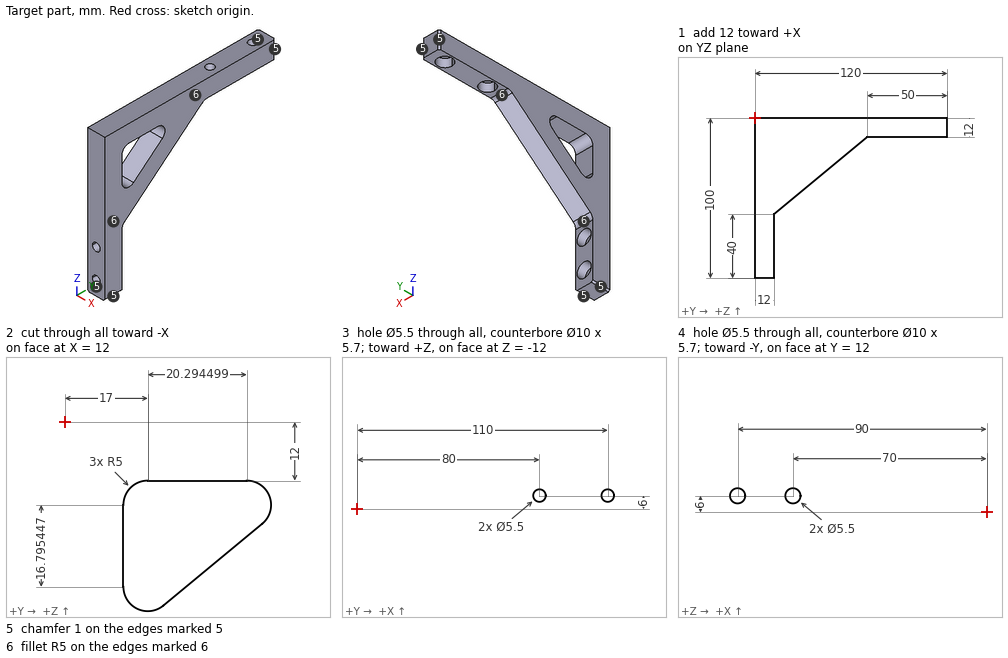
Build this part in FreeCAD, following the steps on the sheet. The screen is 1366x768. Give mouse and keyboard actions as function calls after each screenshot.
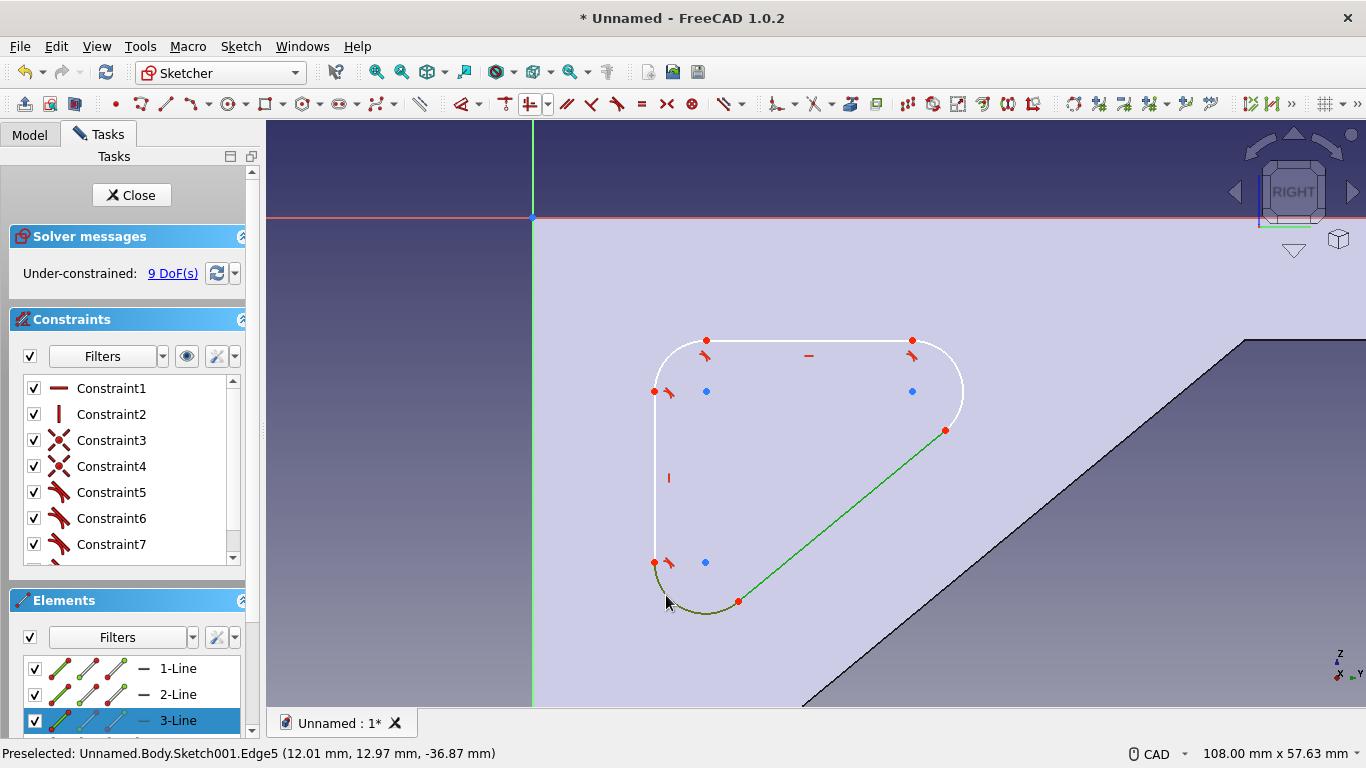
click(617, 104)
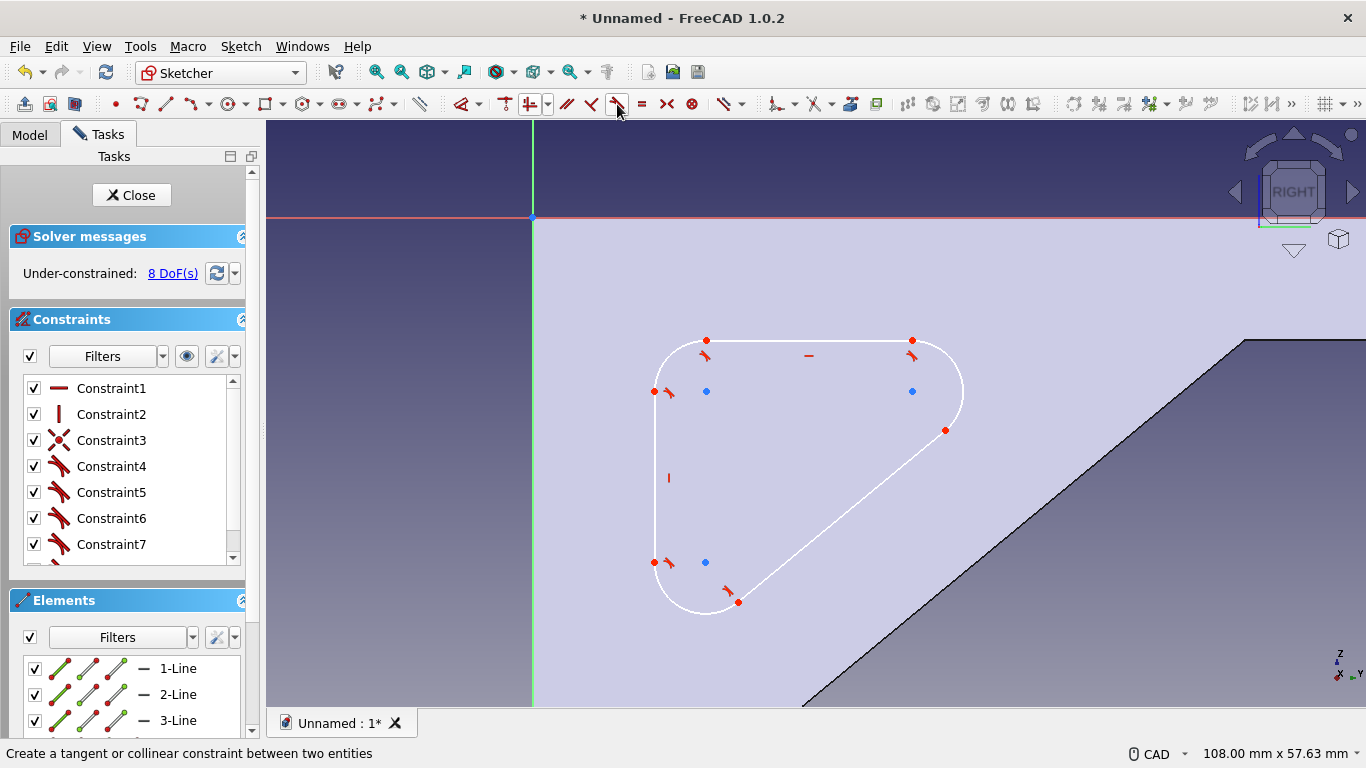
click(800, 551)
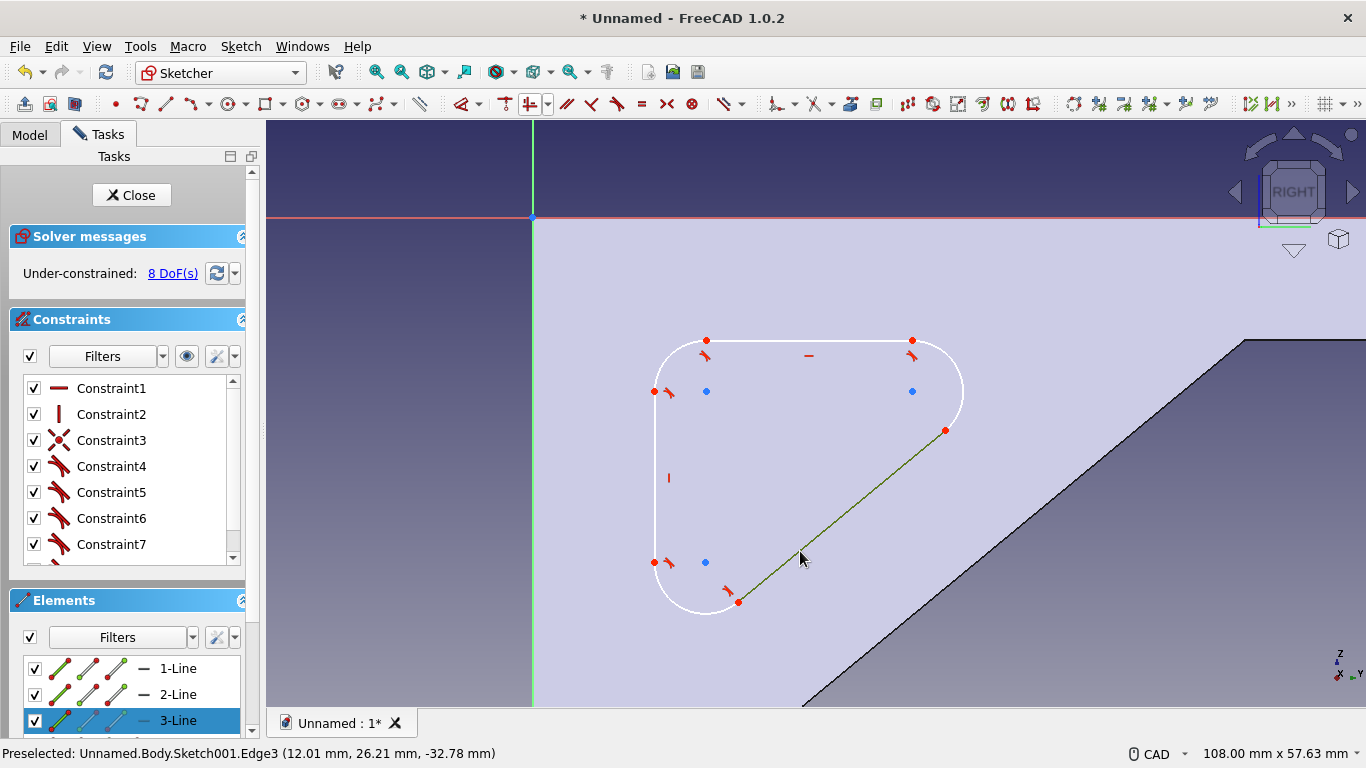
click(963, 399)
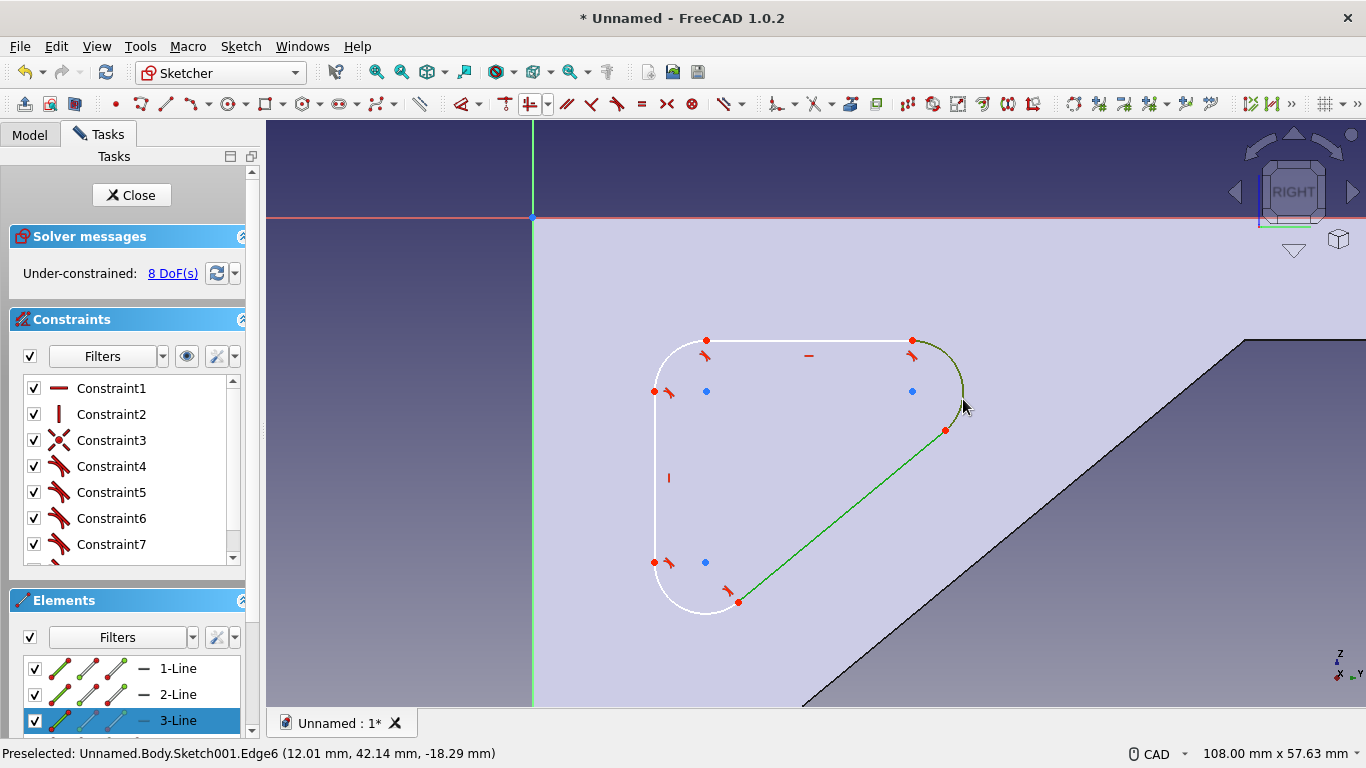
click(617, 104)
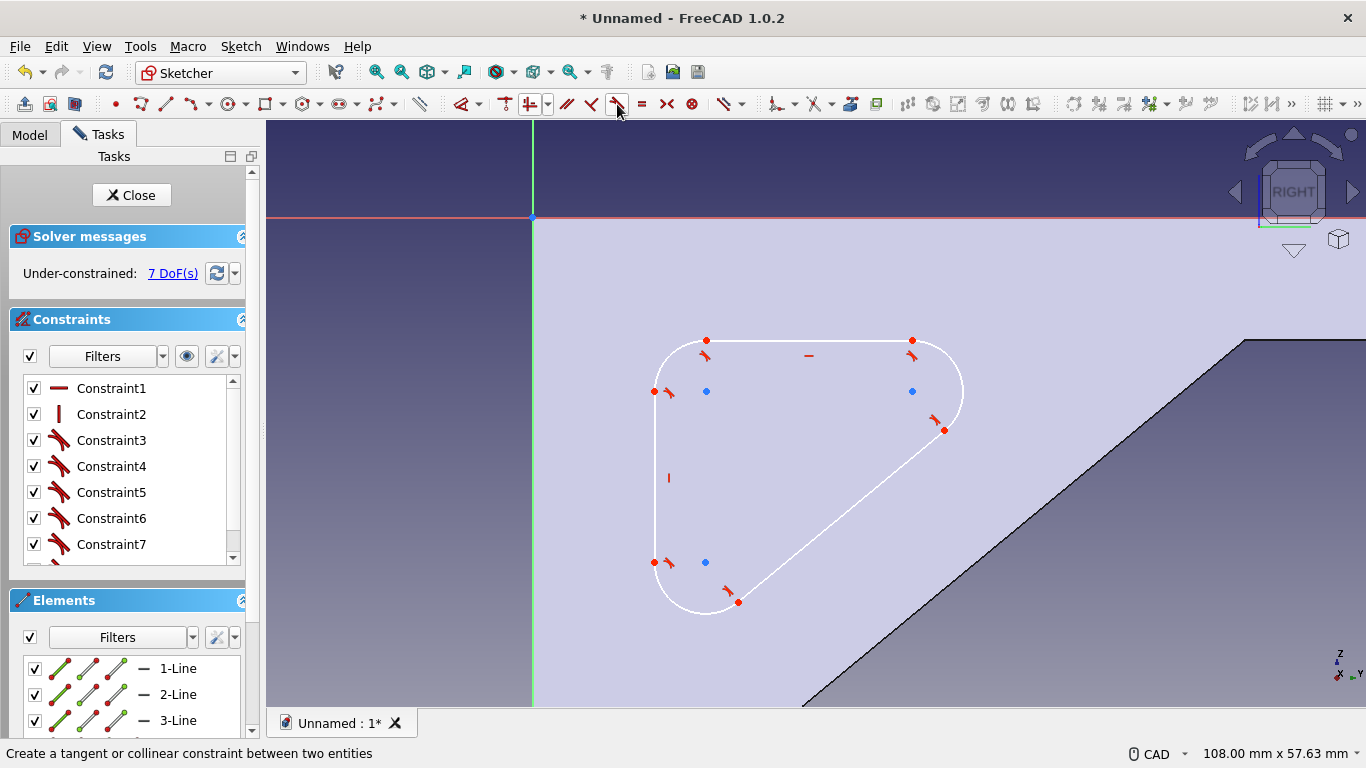
click(683, 346)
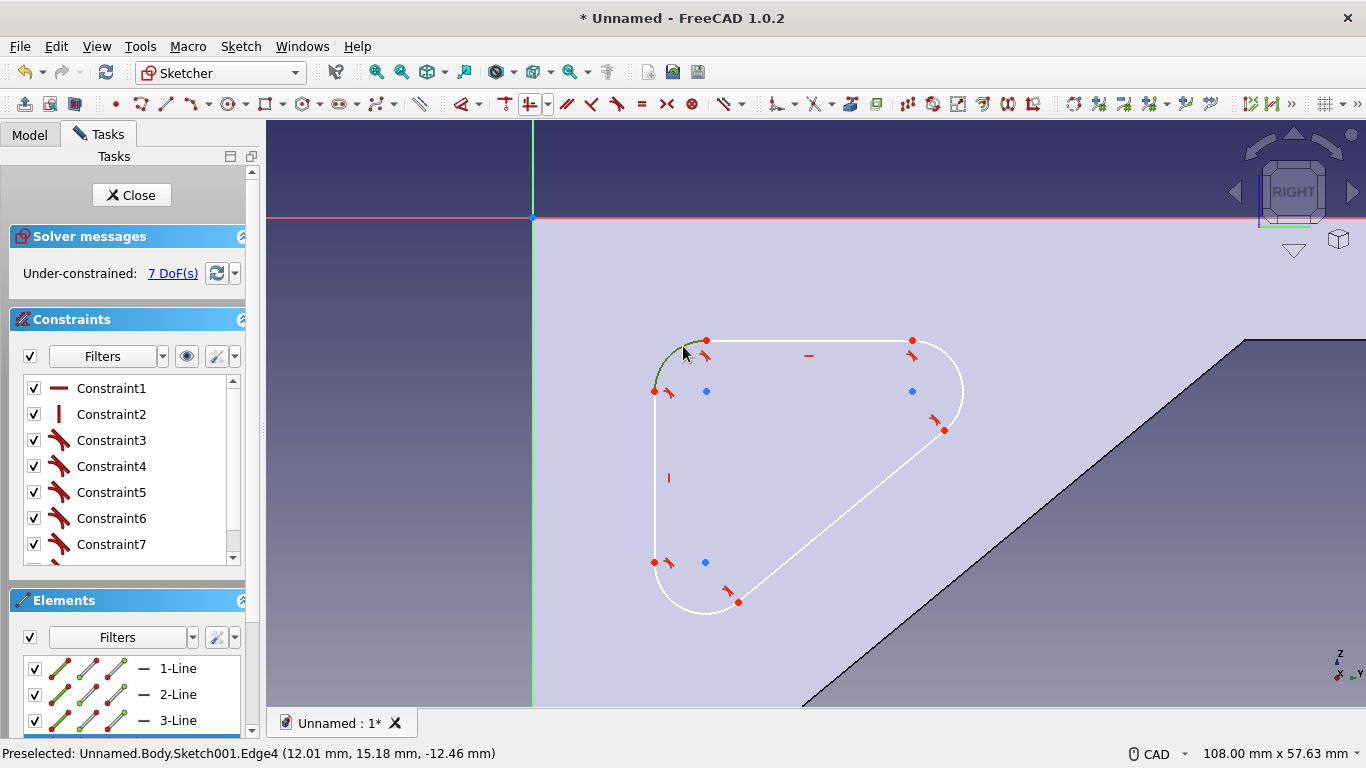
click(666, 595)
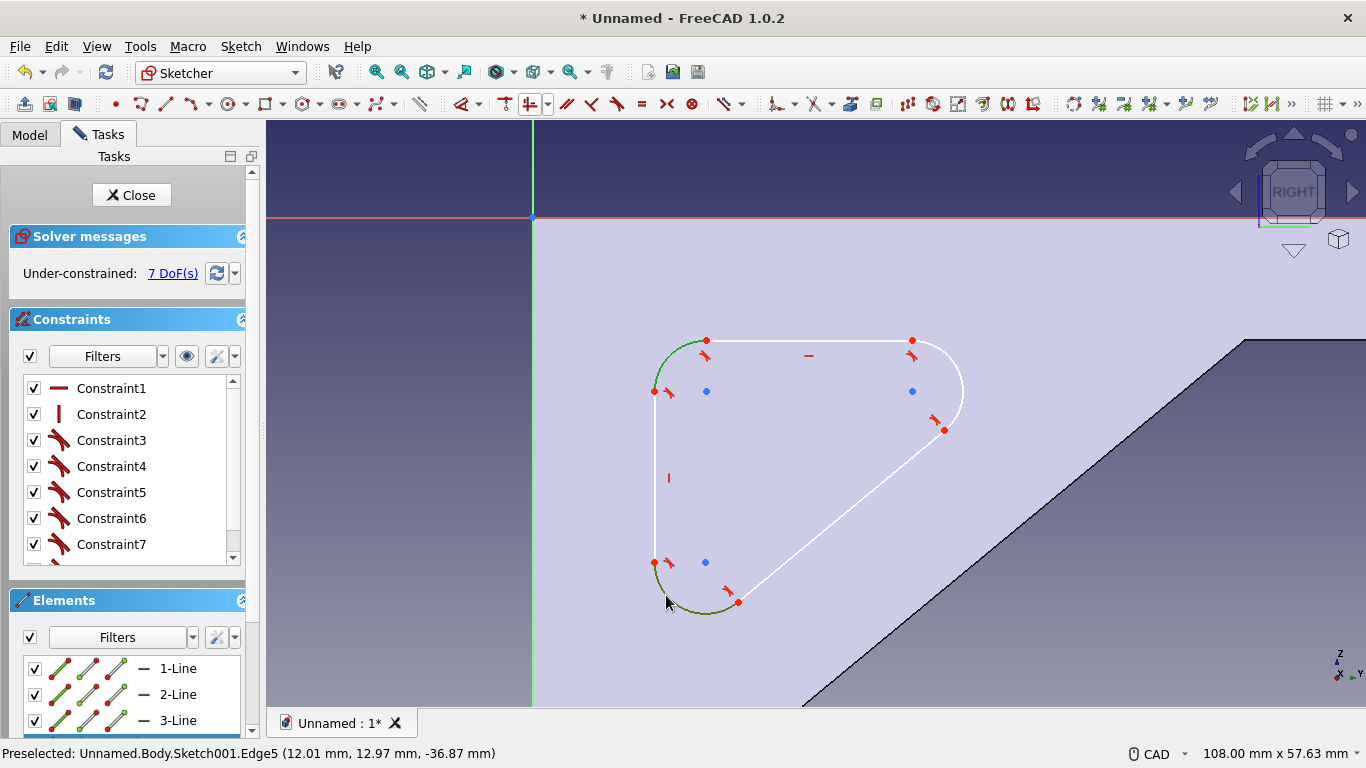
click(962, 399)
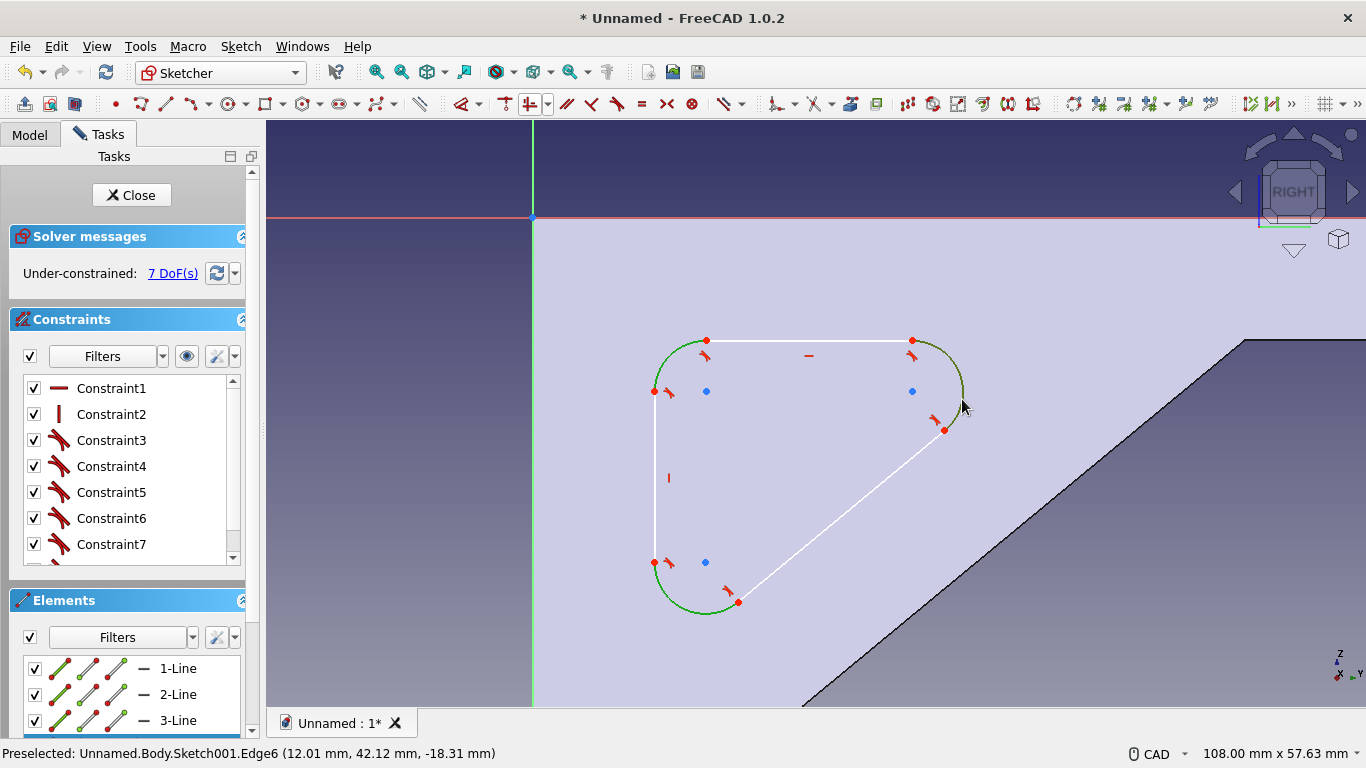
click(642, 104)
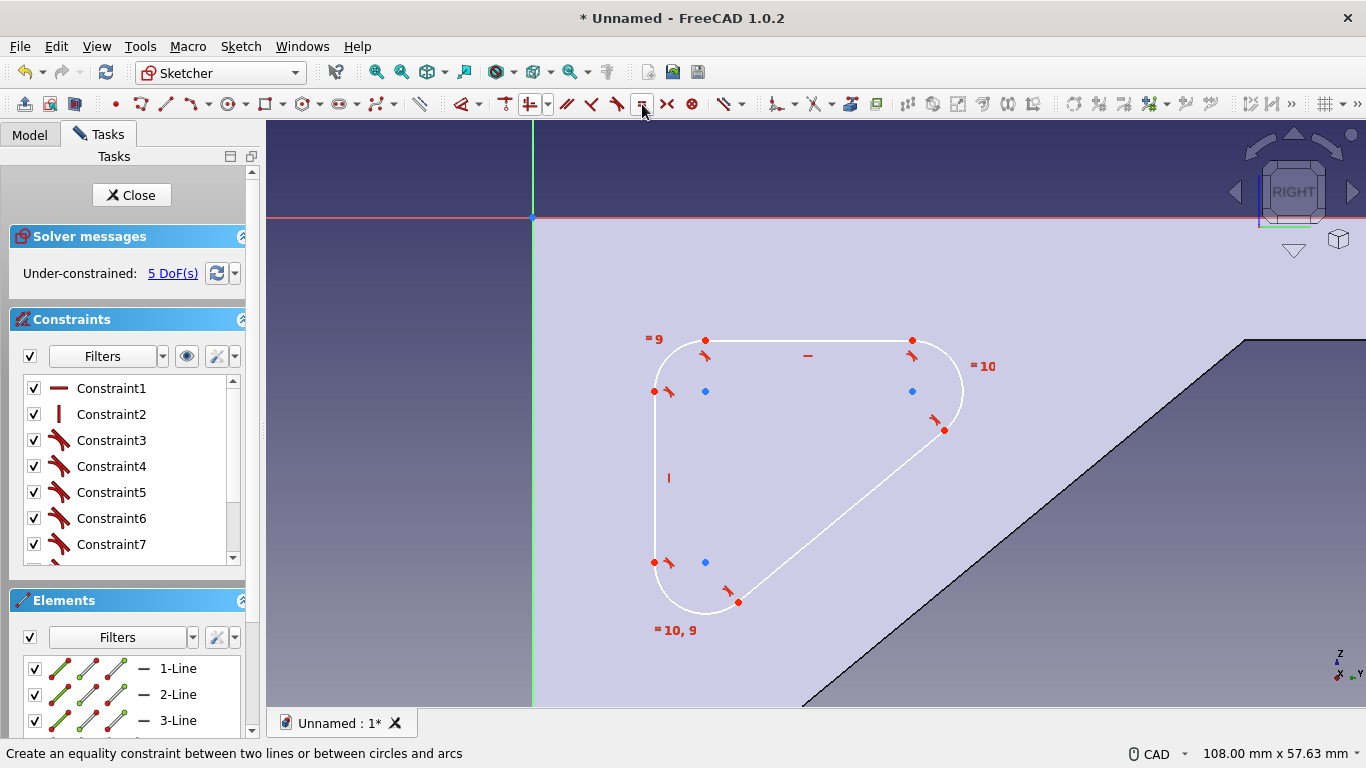
click(460, 104)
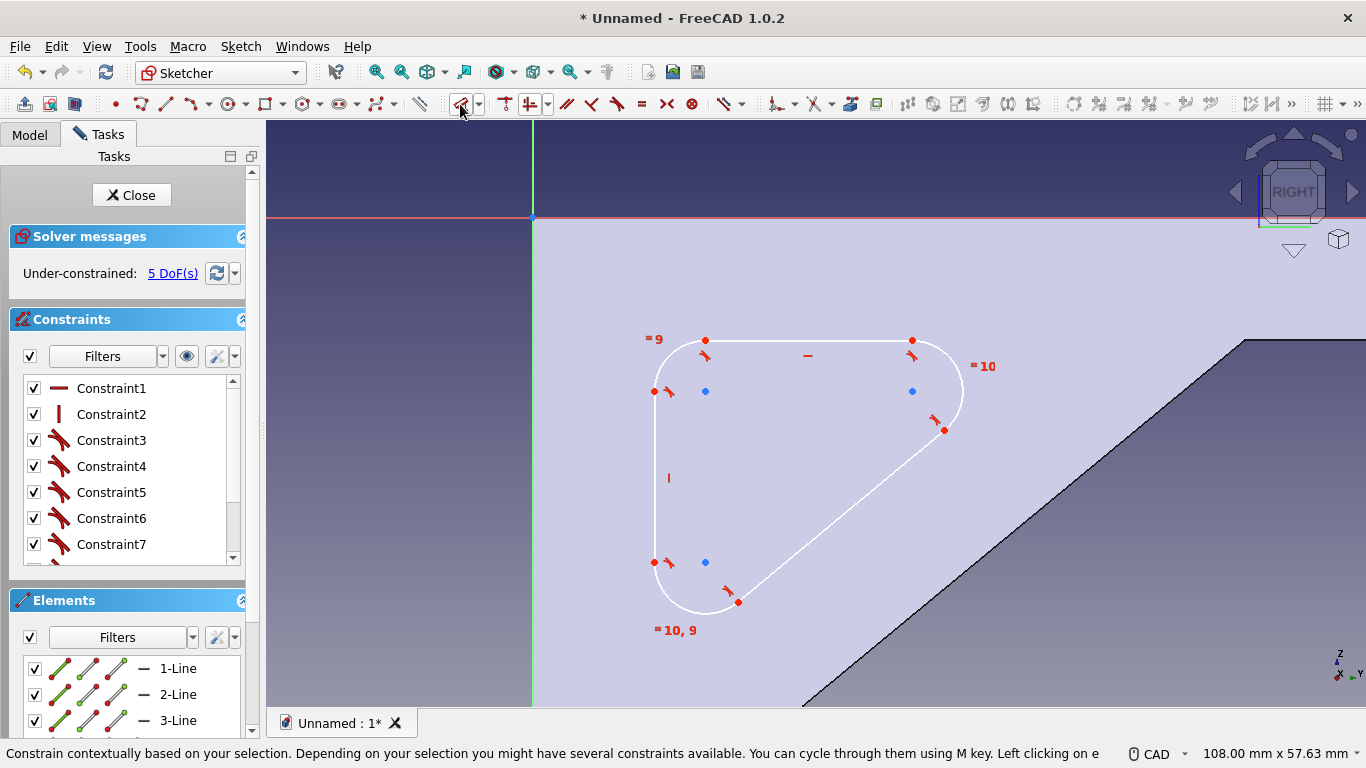
click(683, 346)
click(669, 317)